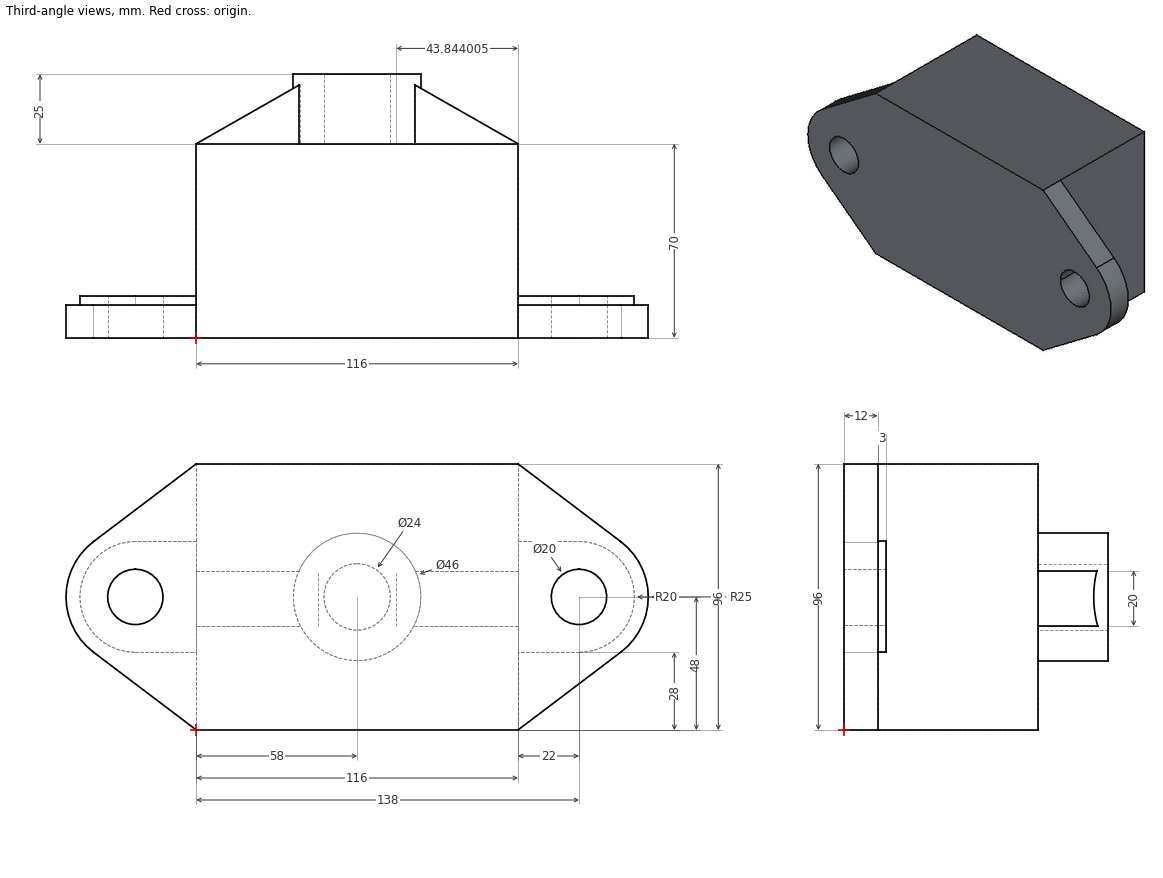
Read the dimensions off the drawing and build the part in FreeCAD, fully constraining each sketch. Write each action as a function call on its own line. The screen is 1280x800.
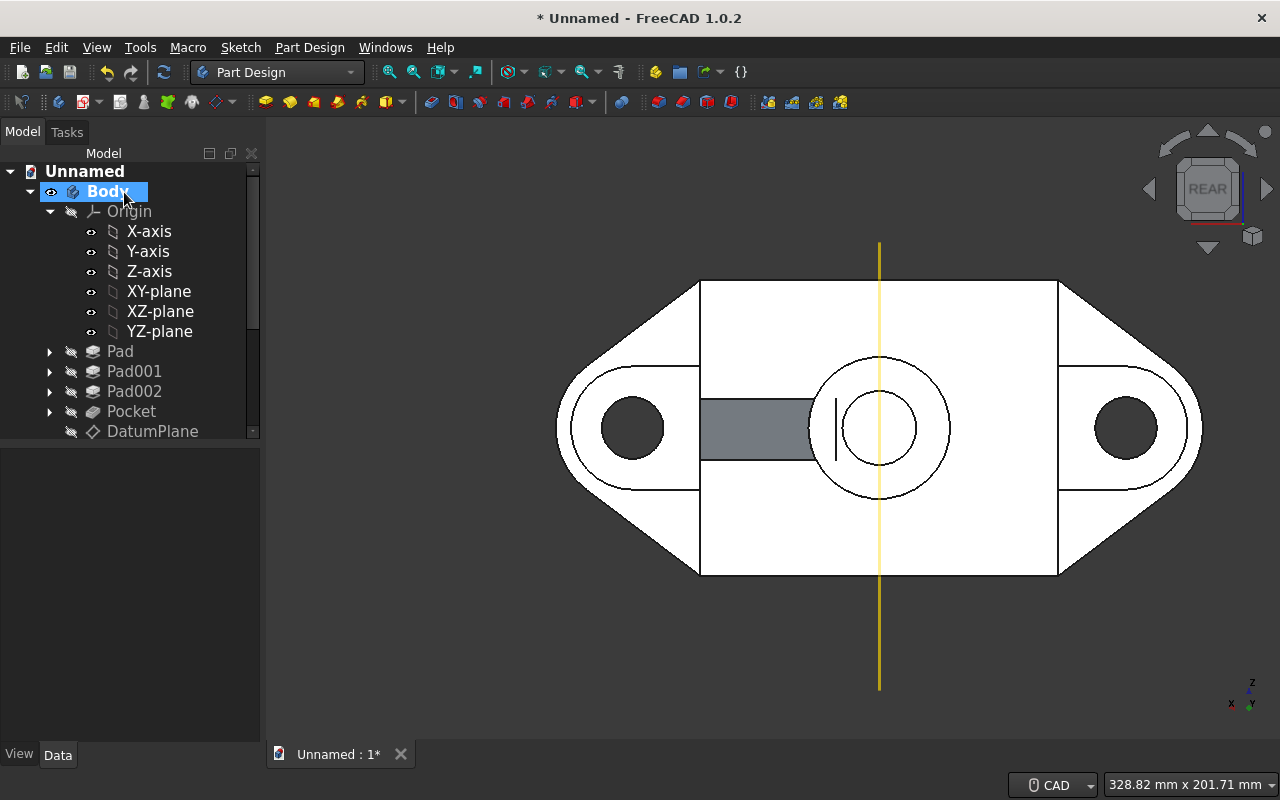
scroll(100, 307, down, 3)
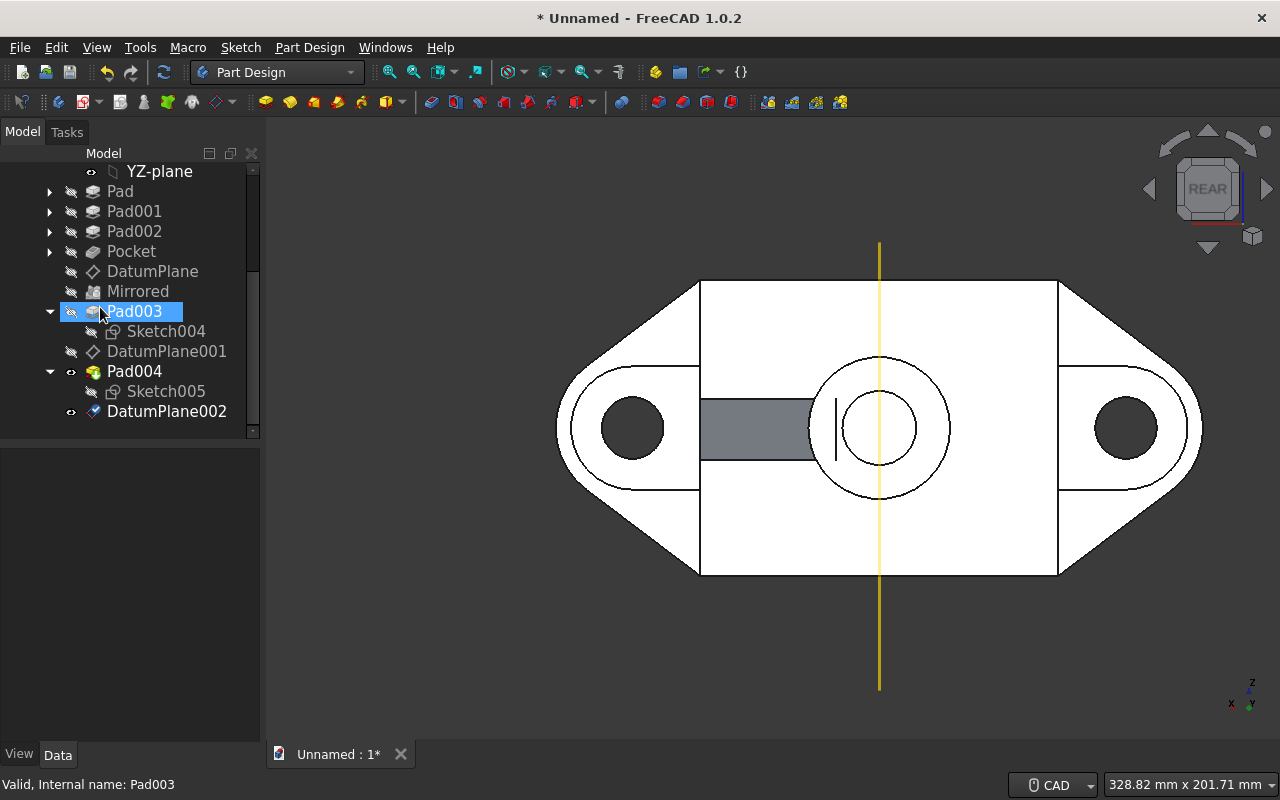
click(116, 372)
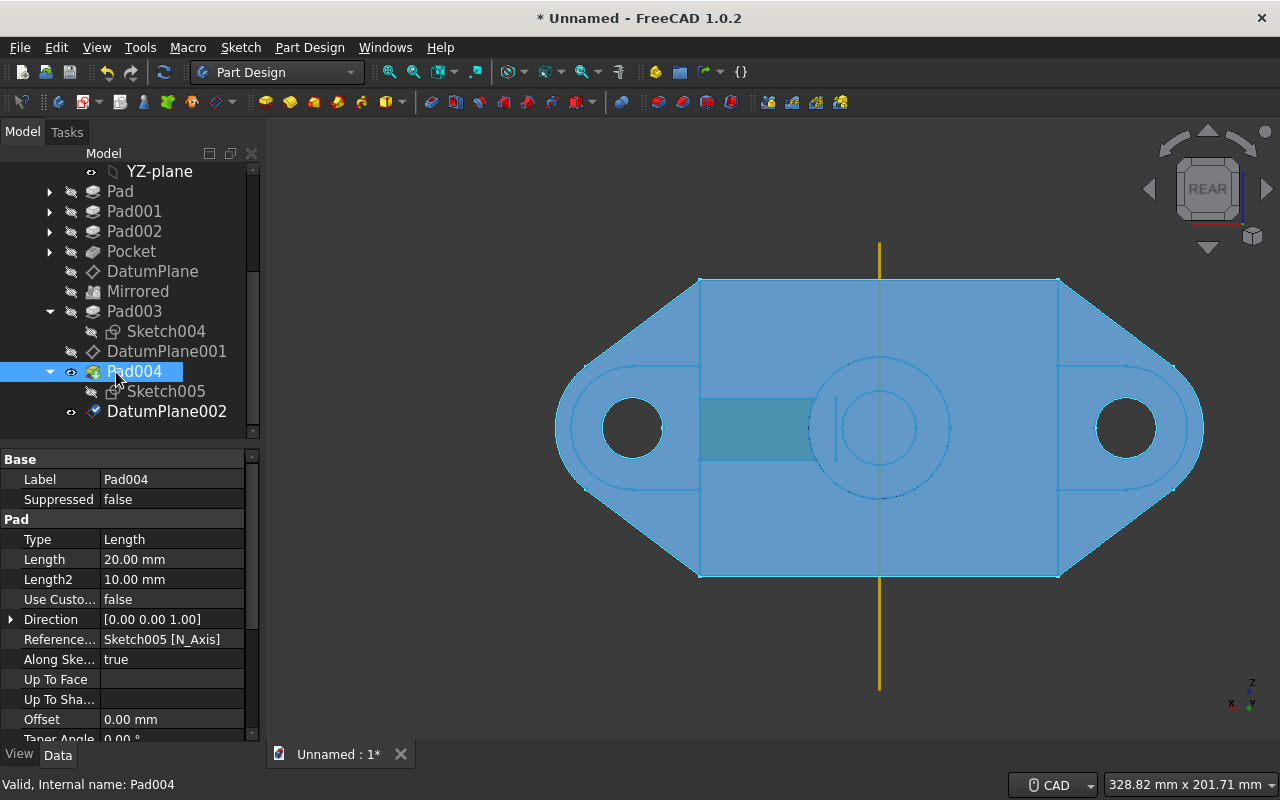
click(768, 102)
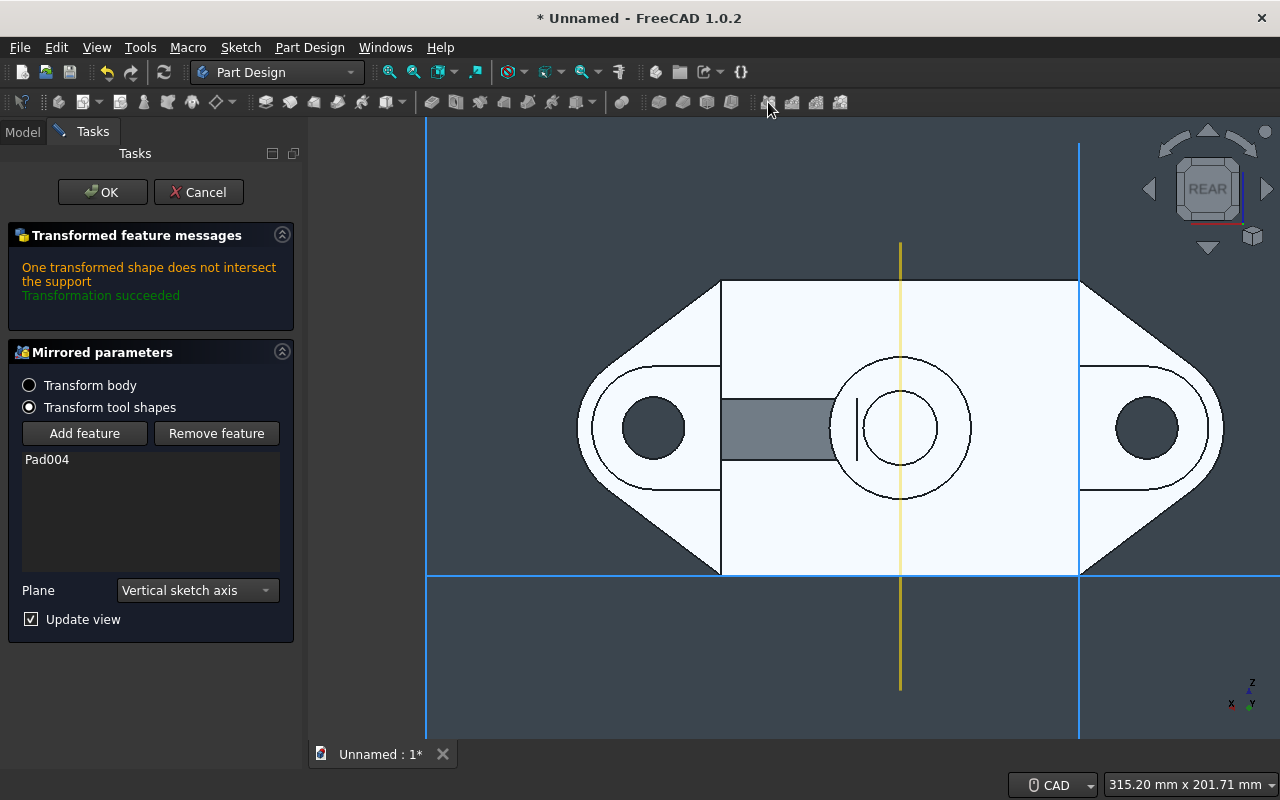
click(198, 590)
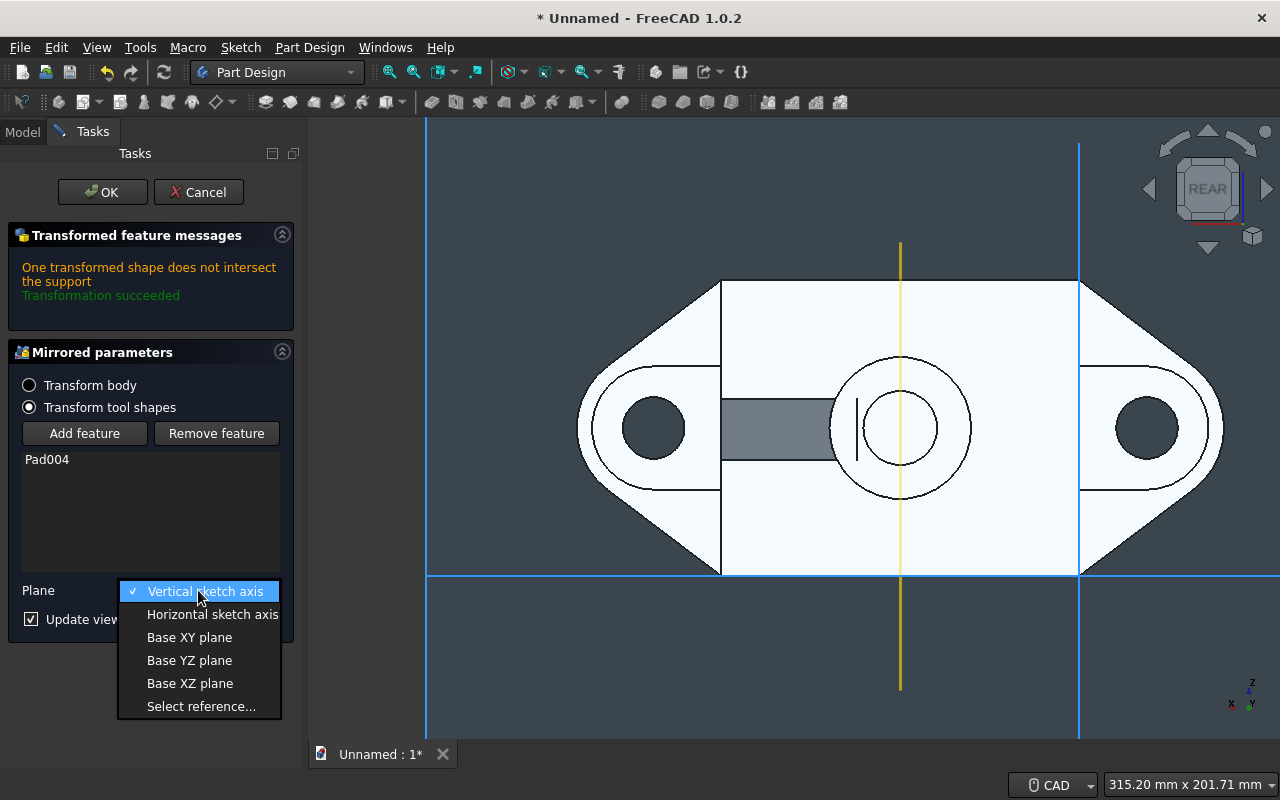
click(198, 706)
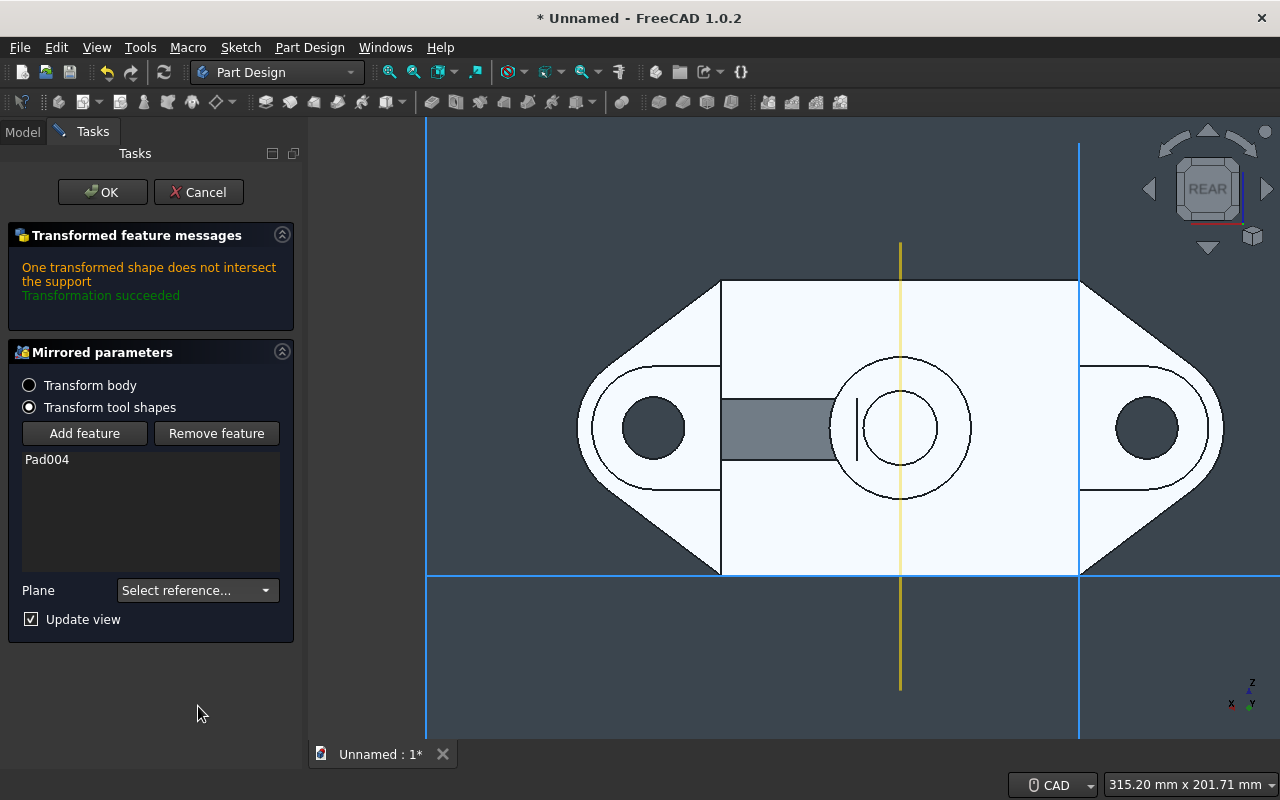
click(23, 131)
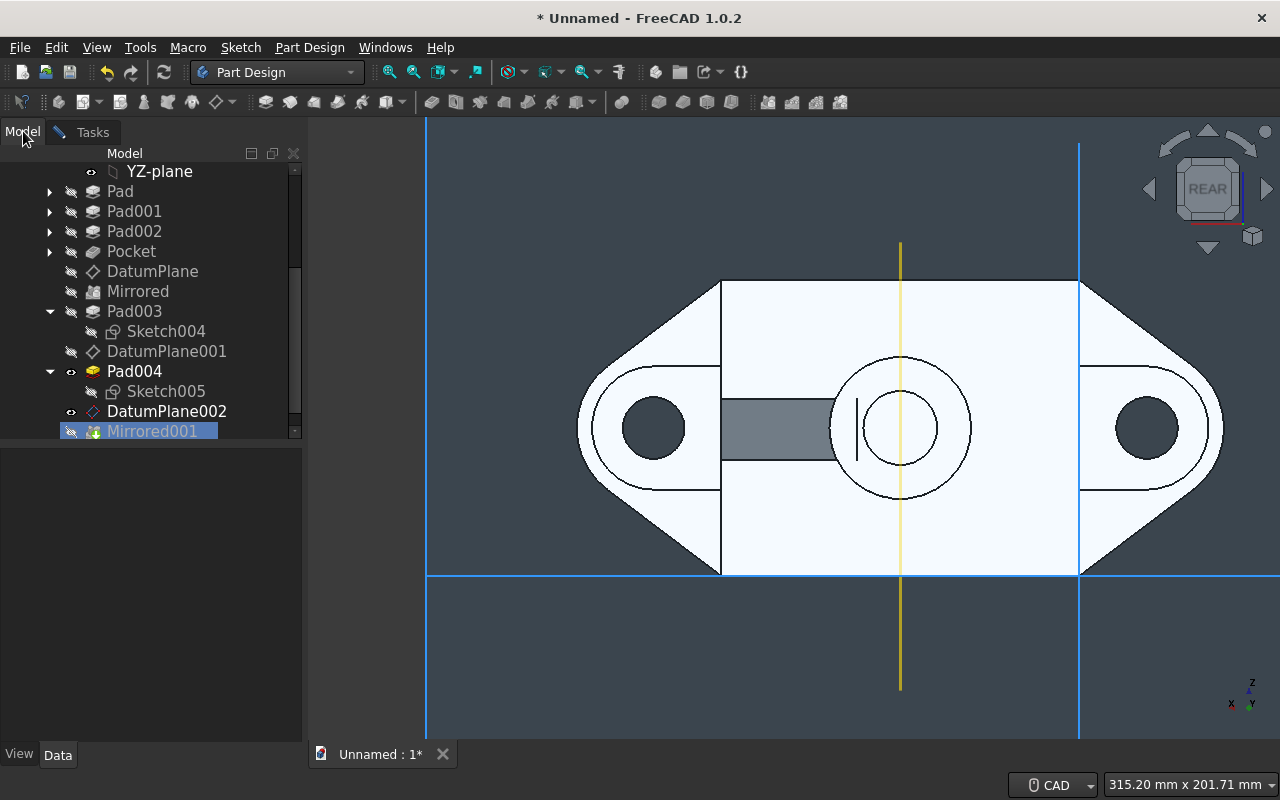
click(116, 412)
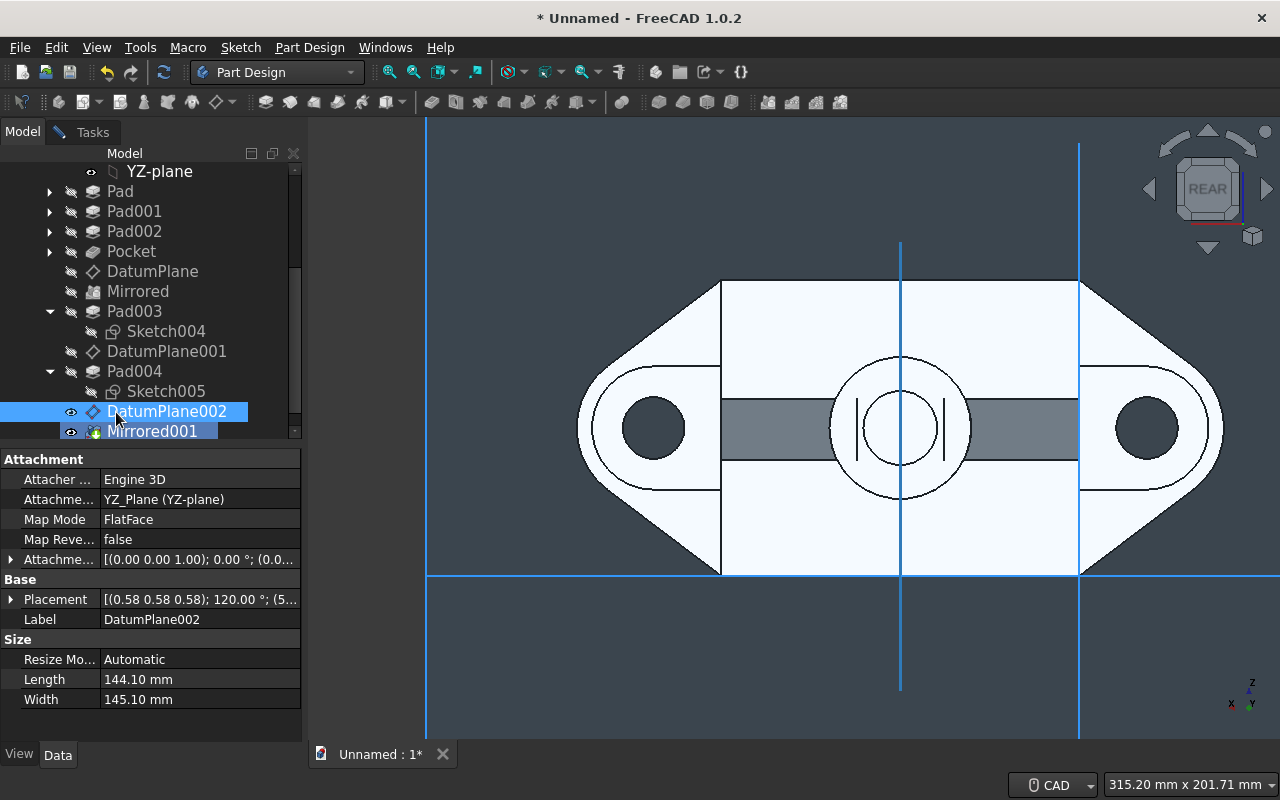
click(84, 131)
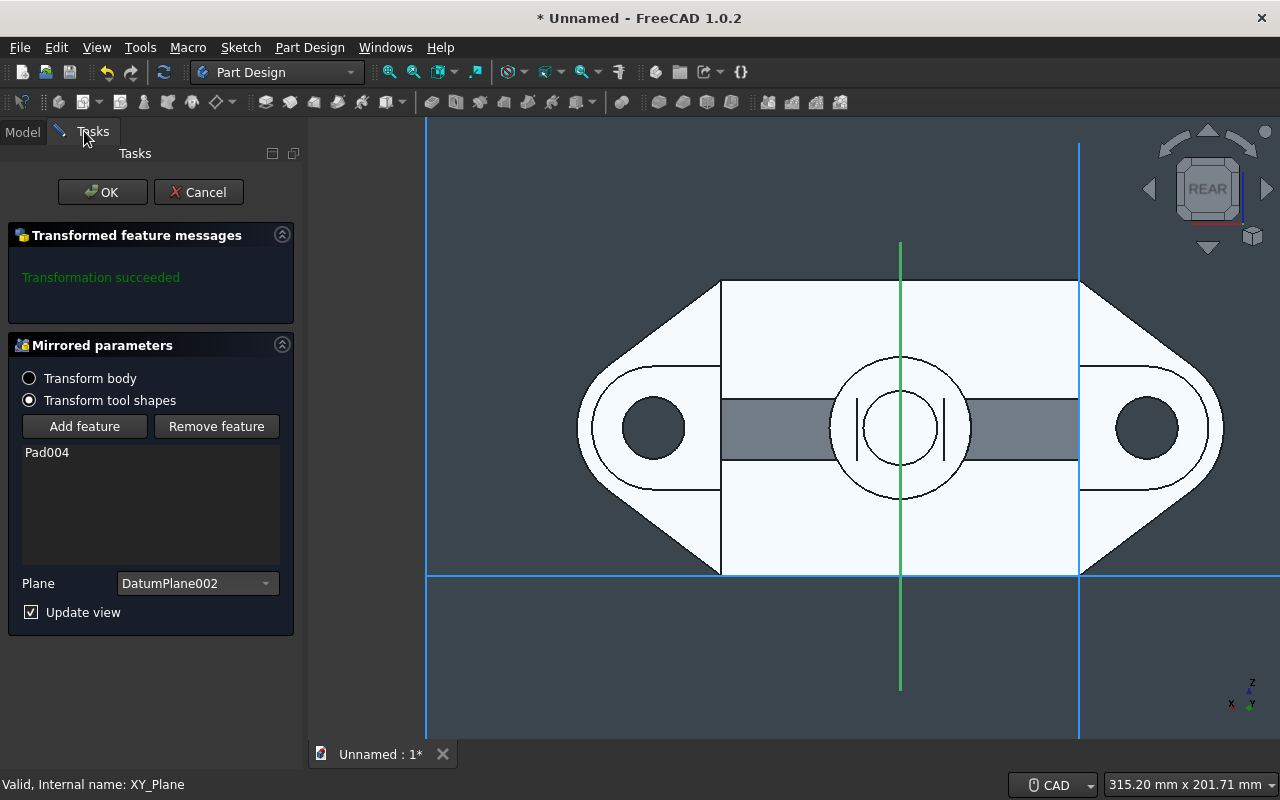
click(103, 192)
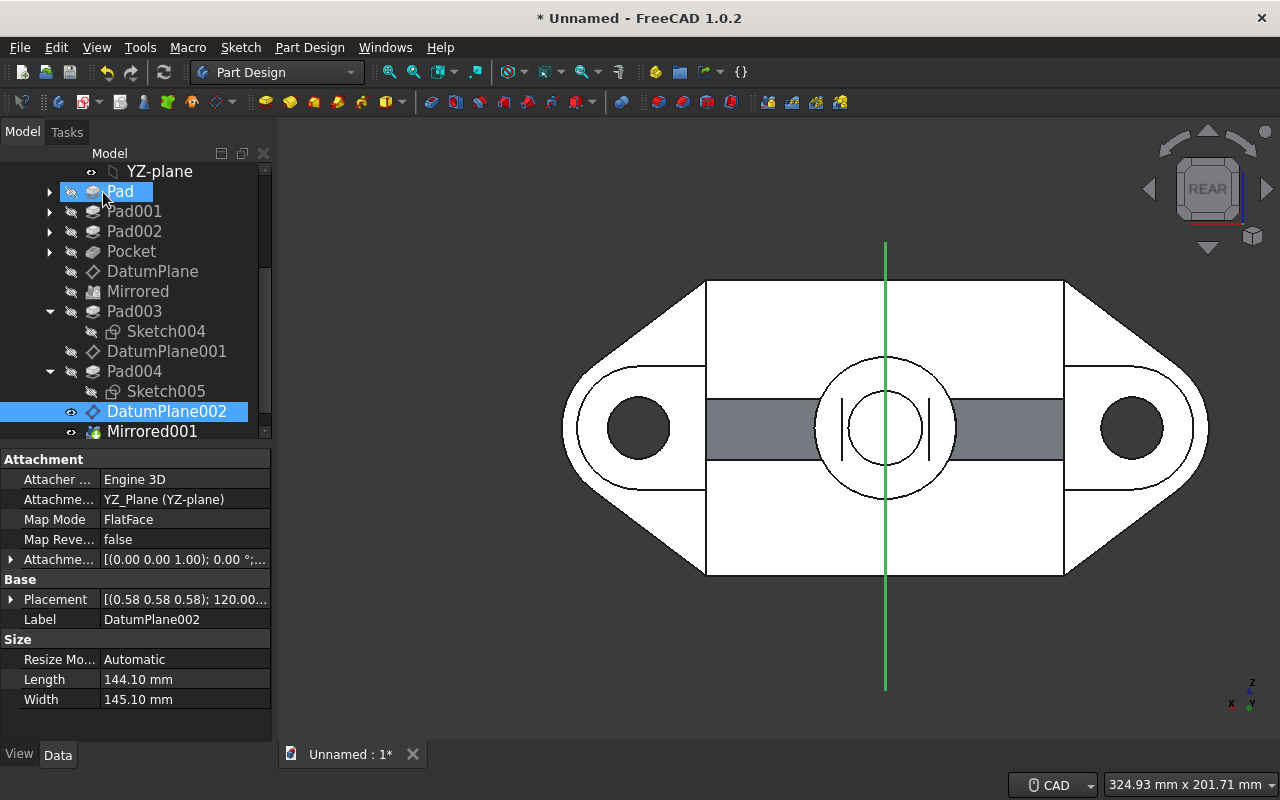
click(116, 412)
key(space)